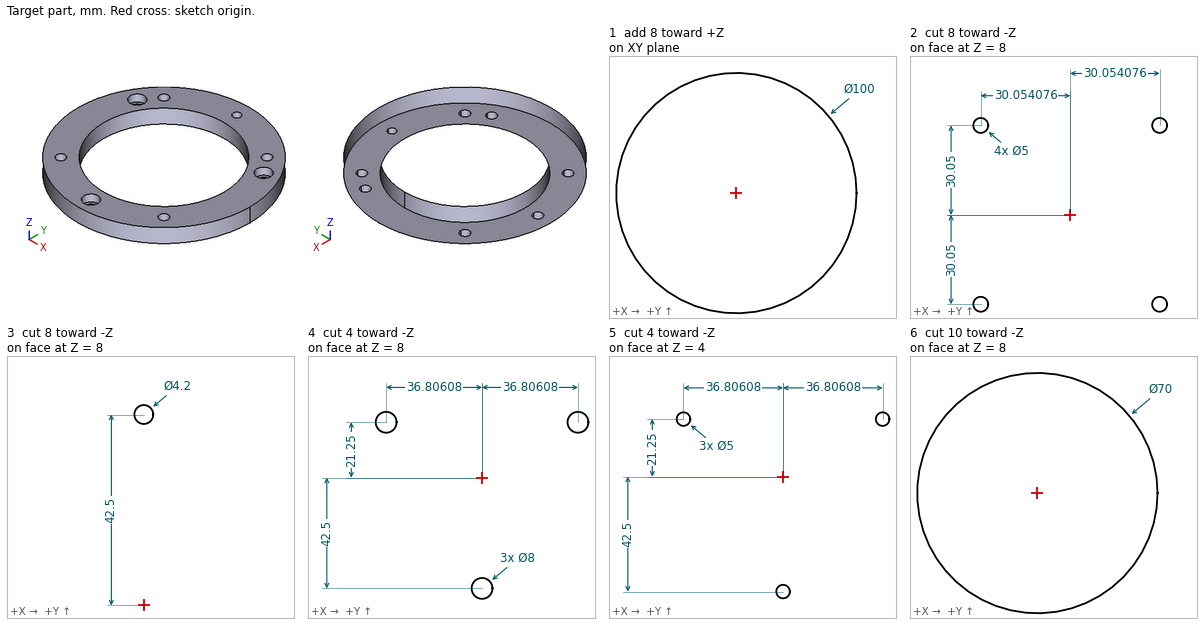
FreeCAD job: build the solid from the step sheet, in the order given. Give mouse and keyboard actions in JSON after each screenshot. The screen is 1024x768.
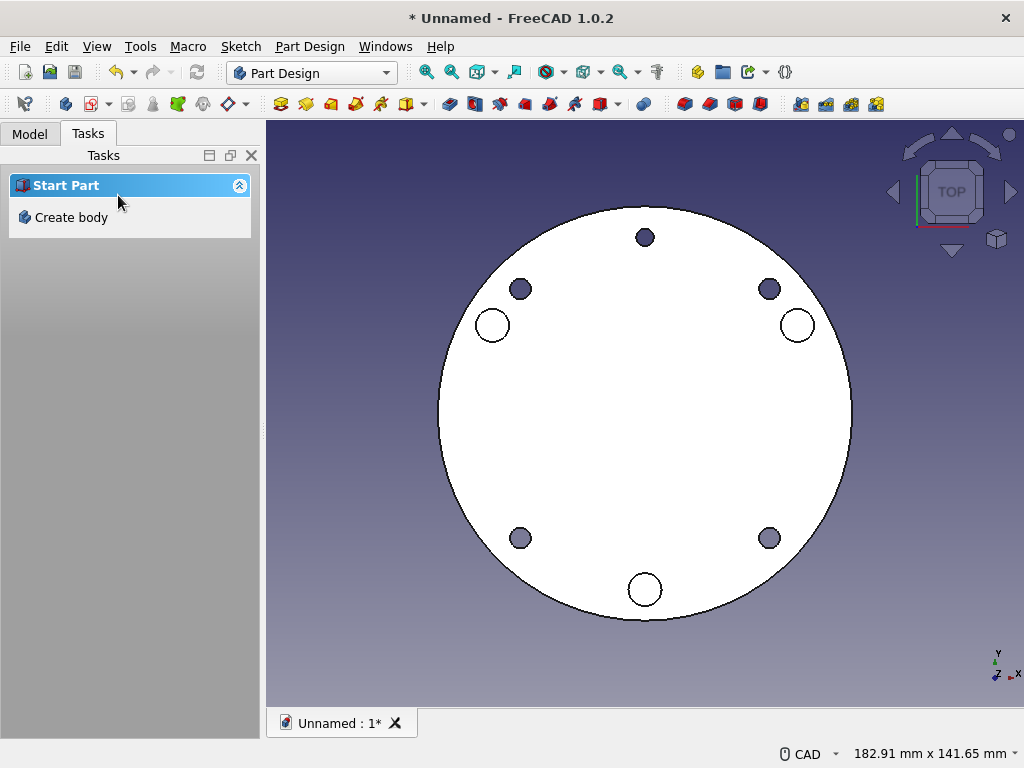
{"action": "left_click", "coordinate": [798, 324]}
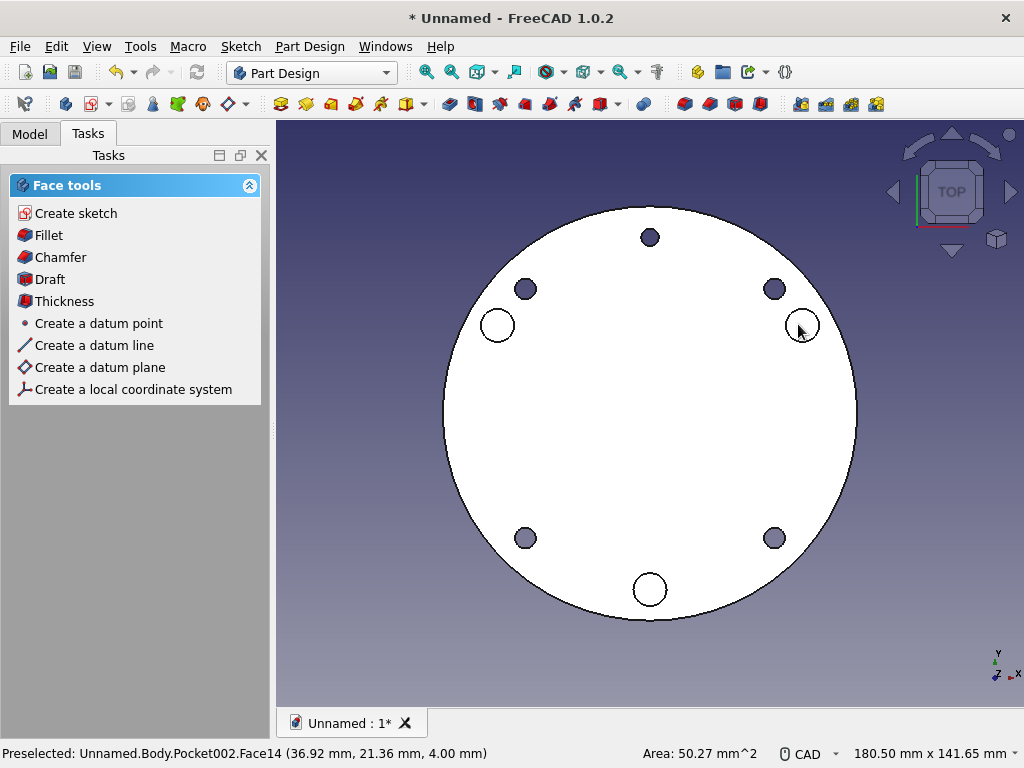
{"action": "left_click", "coordinate": [90, 104]}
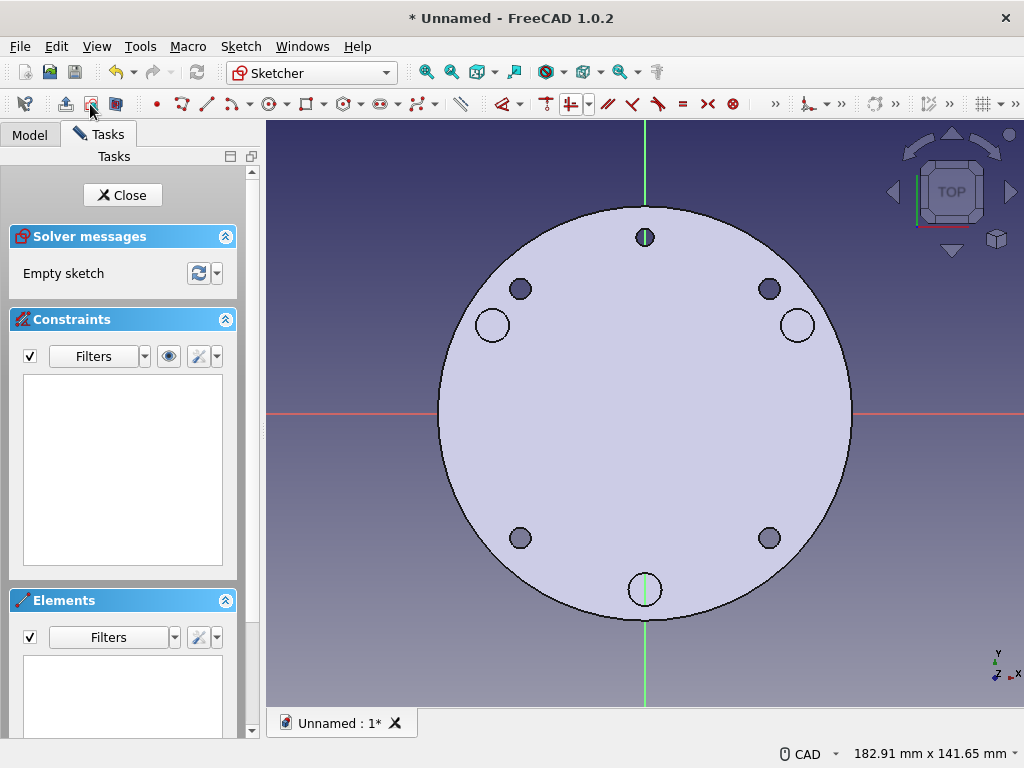
{"action": "left_click", "coordinate": [116, 104]}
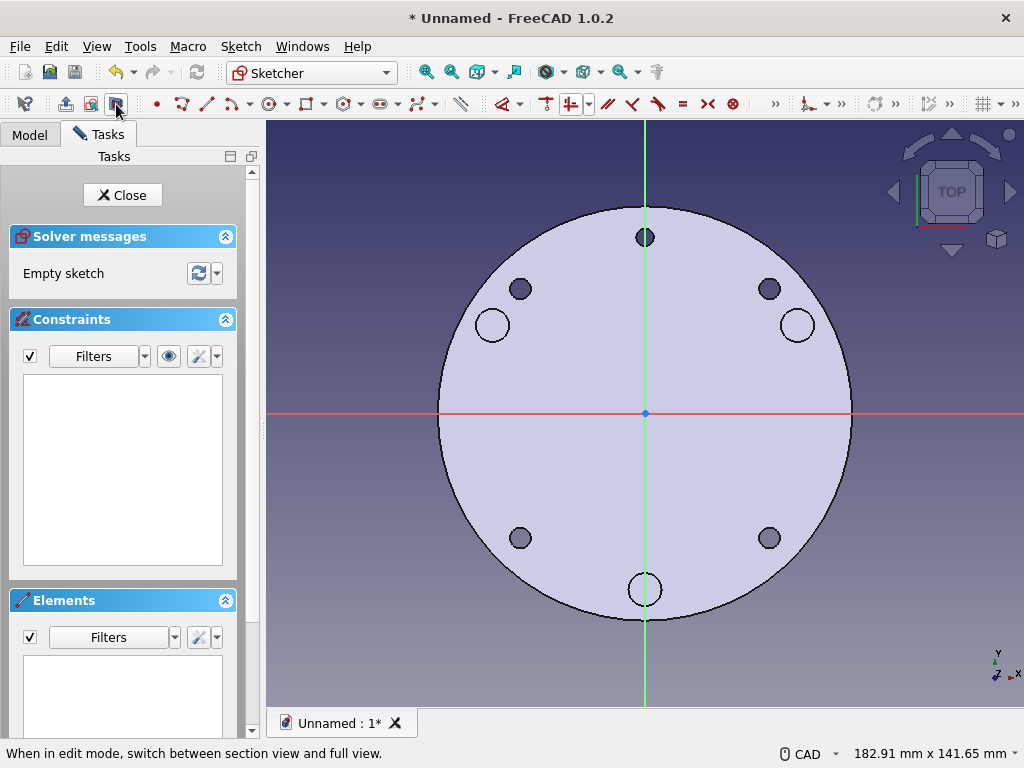
{"action": "left_click", "coordinate": [268, 104]}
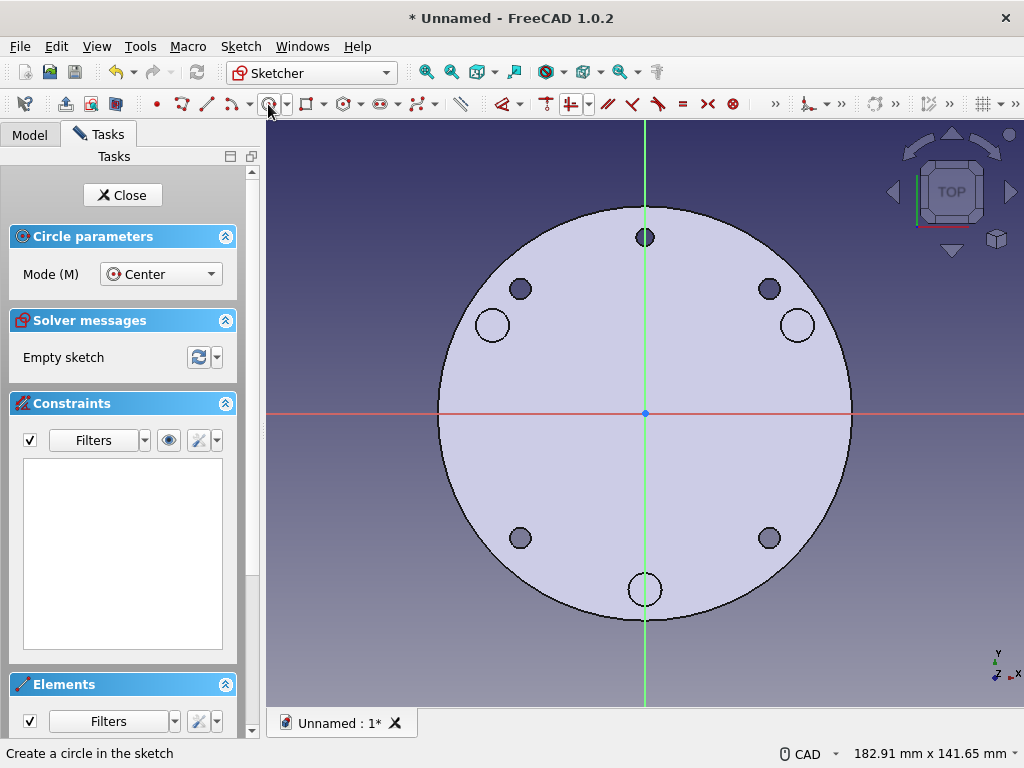
{"action": "scroll", "coordinate": [492, 325], "scroll_direction": "up", "scroll_amount": 4}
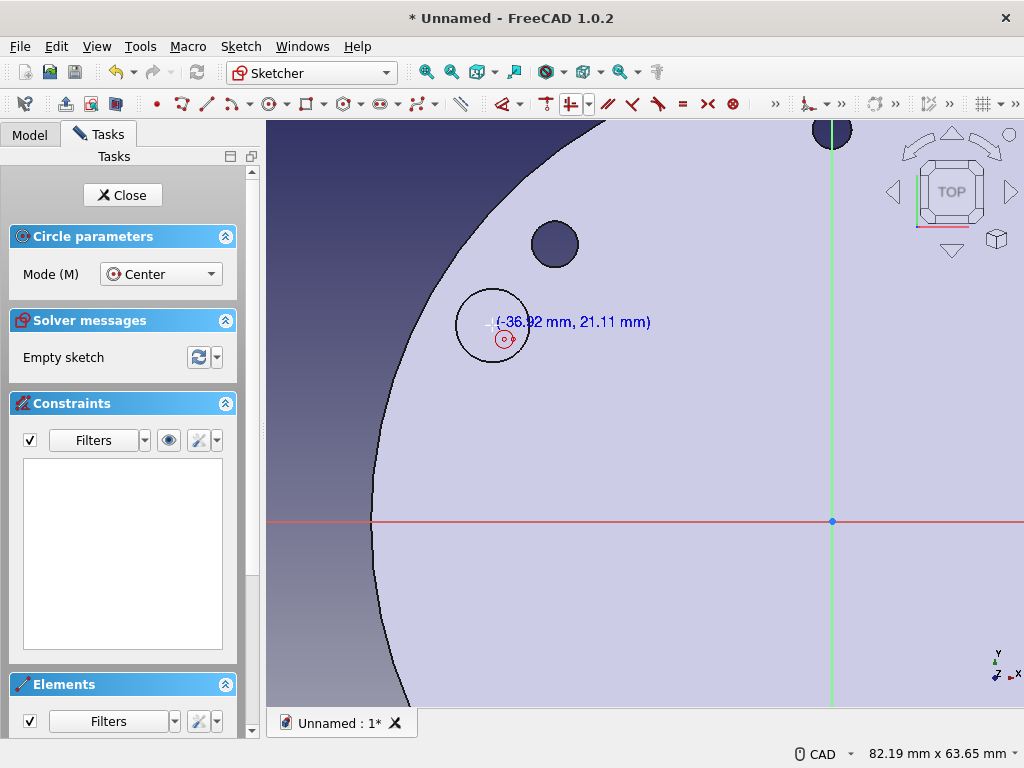
{"action": "left_click", "coordinate": [493, 326]}
{"action": "mouse_move", "coordinate": [509, 309]}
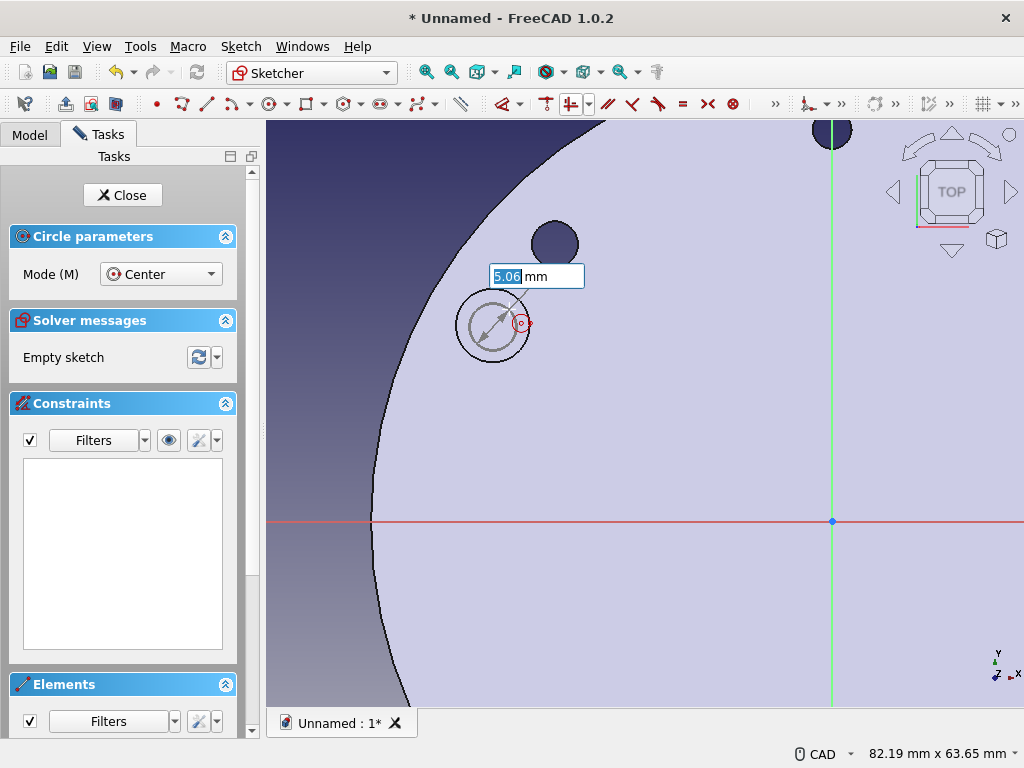
{"action": "type", "text": "5"}
{"action": "key", "text": "Return"}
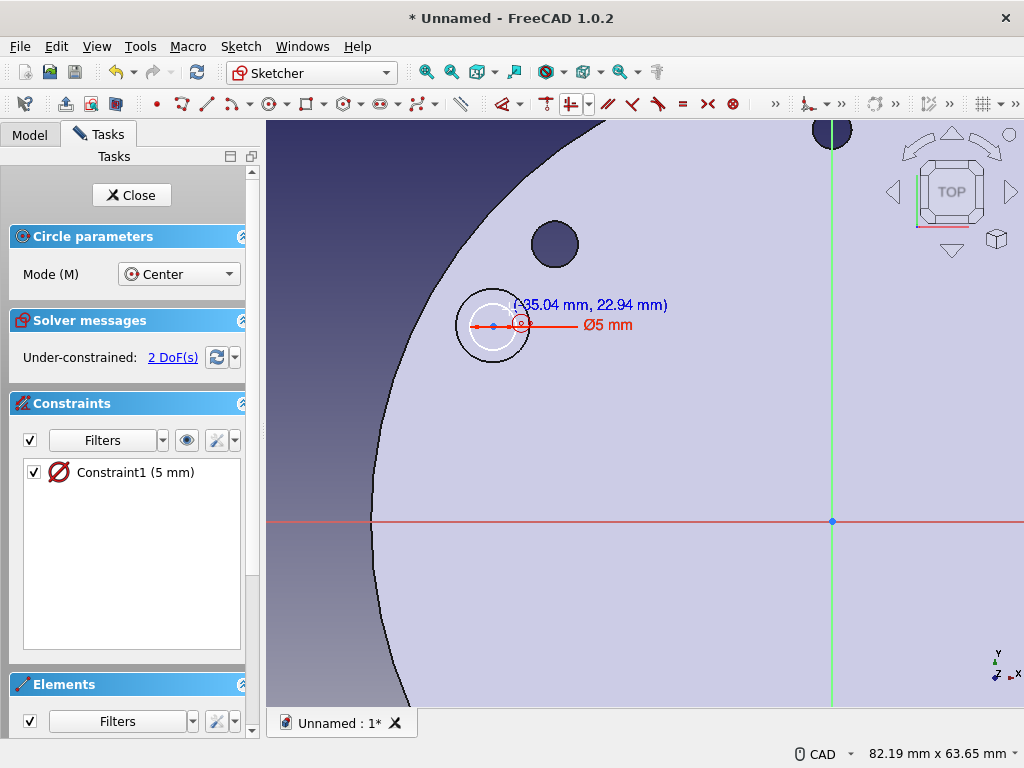
{"action": "scroll", "coordinate": [294, 163], "scroll_direction": "down", "scroll_amount": 3}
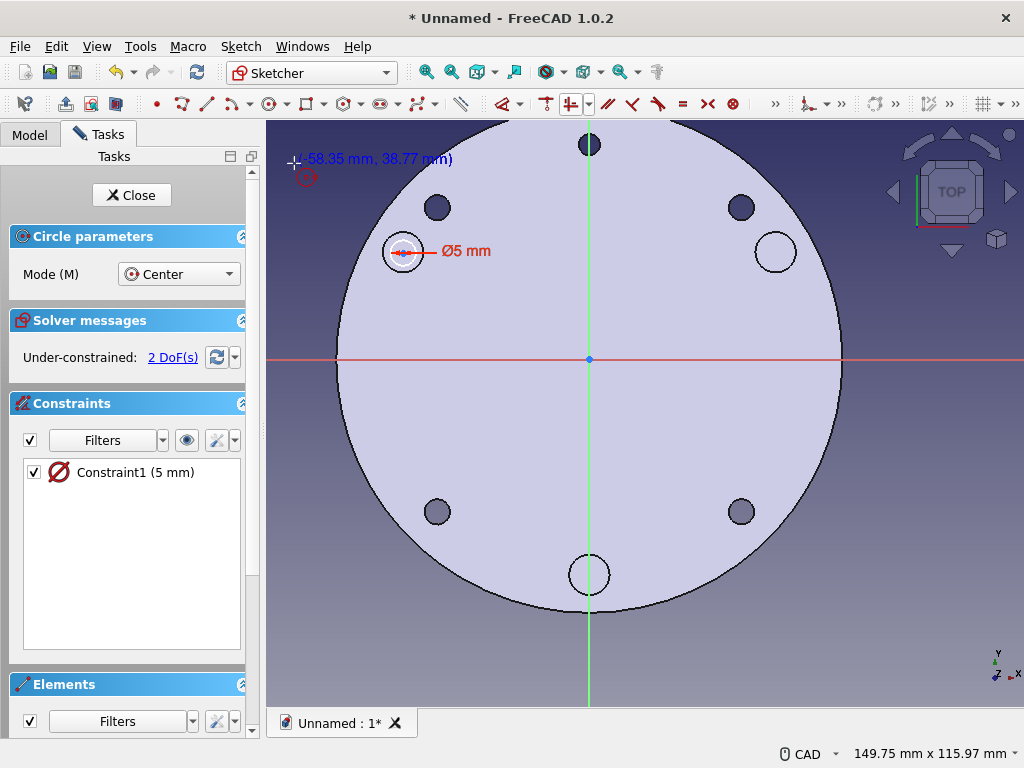
{"action": "scroll", "coordinate": [589, 575], "scroll_direction": "up", "scroll_amount": 3}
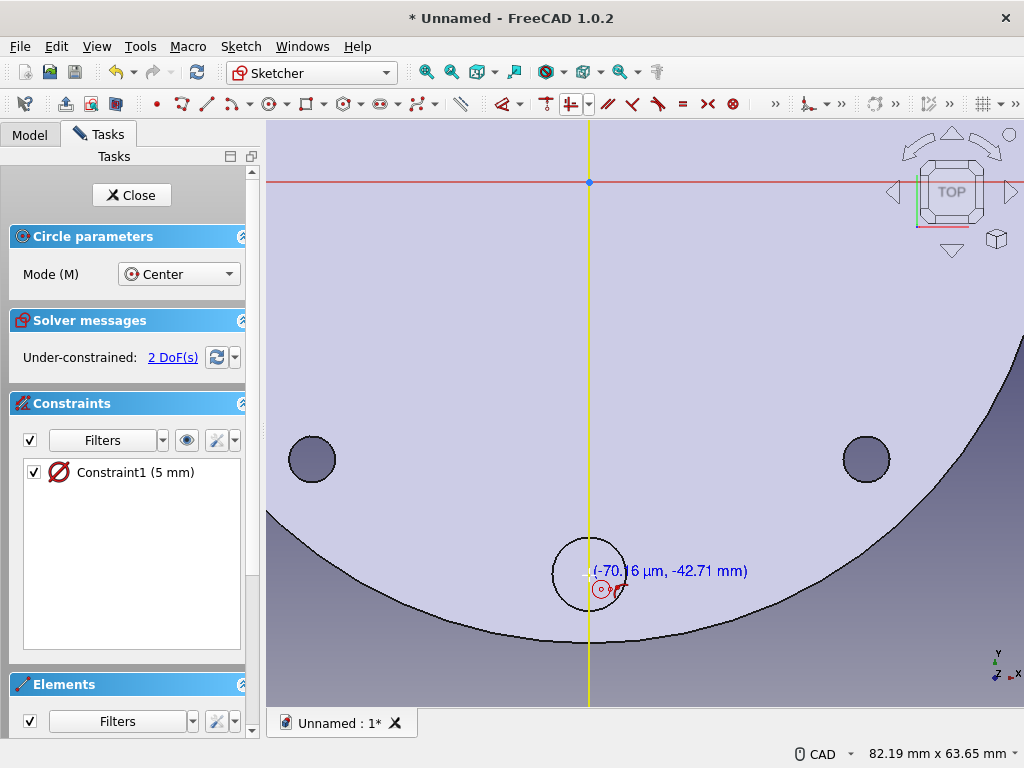
{"action": "left_click", "coordinate": [589, 574]}
{"action": "mouse_move", "coordinate": [606, 558]}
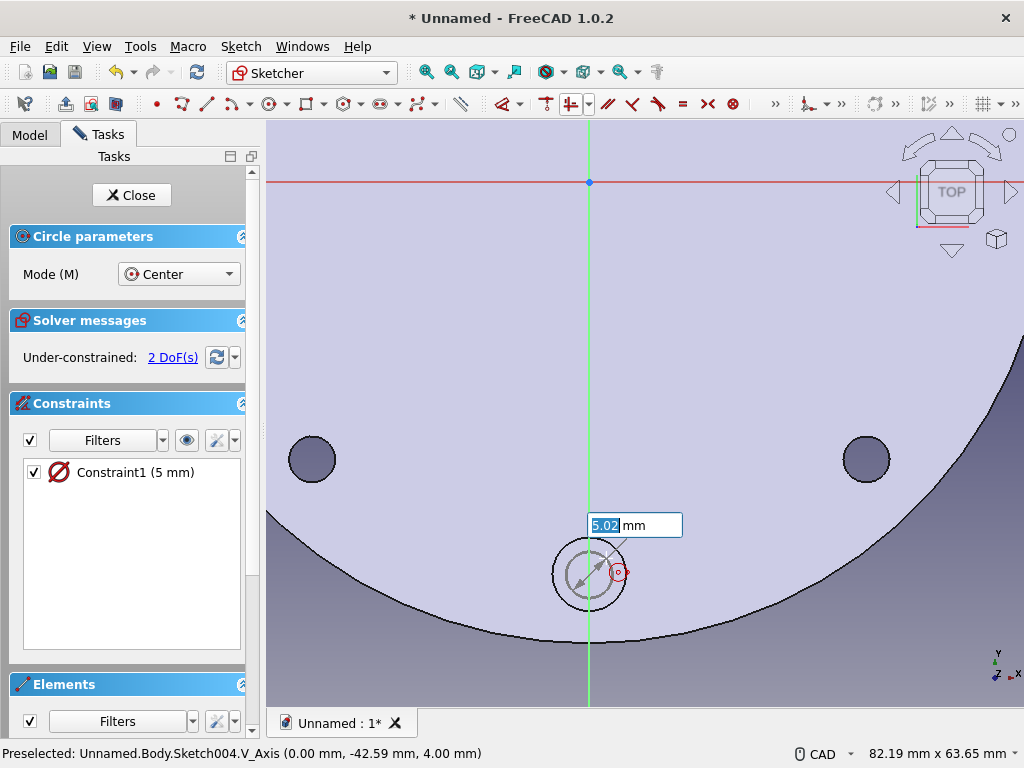
{"action": "type", "text": "5"}
{"action": "key", "text": "Return"}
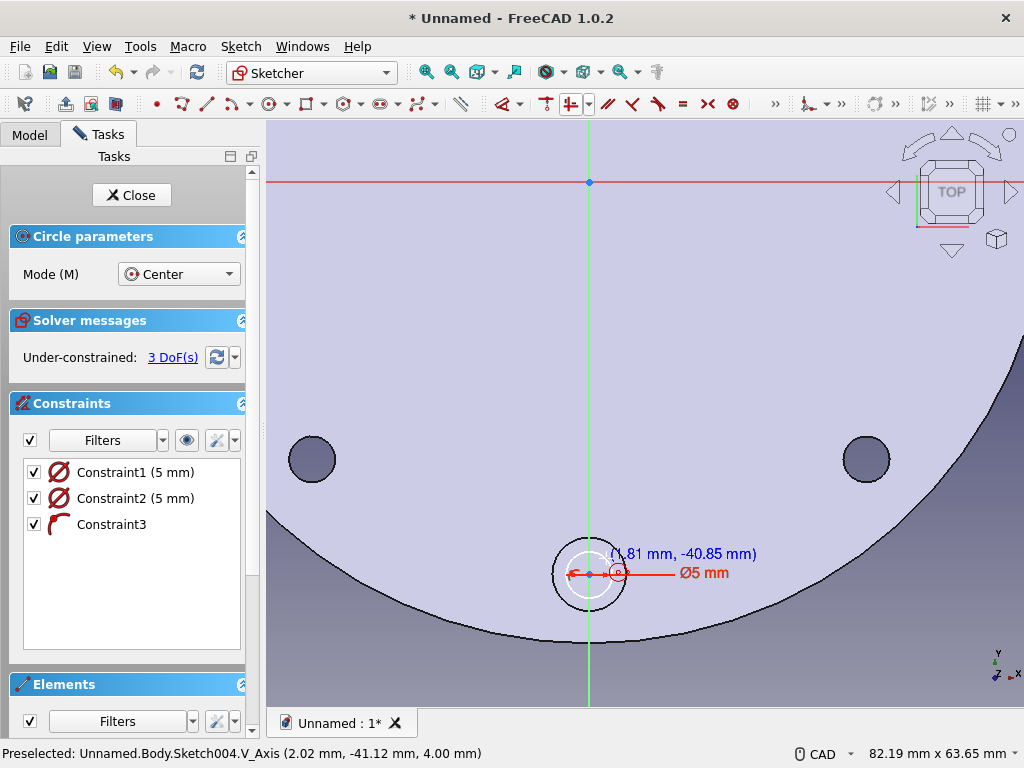
{"action": "scroll", "coordinate": [561, 576], "scroll_direction": "down", "scroll_amount": 3}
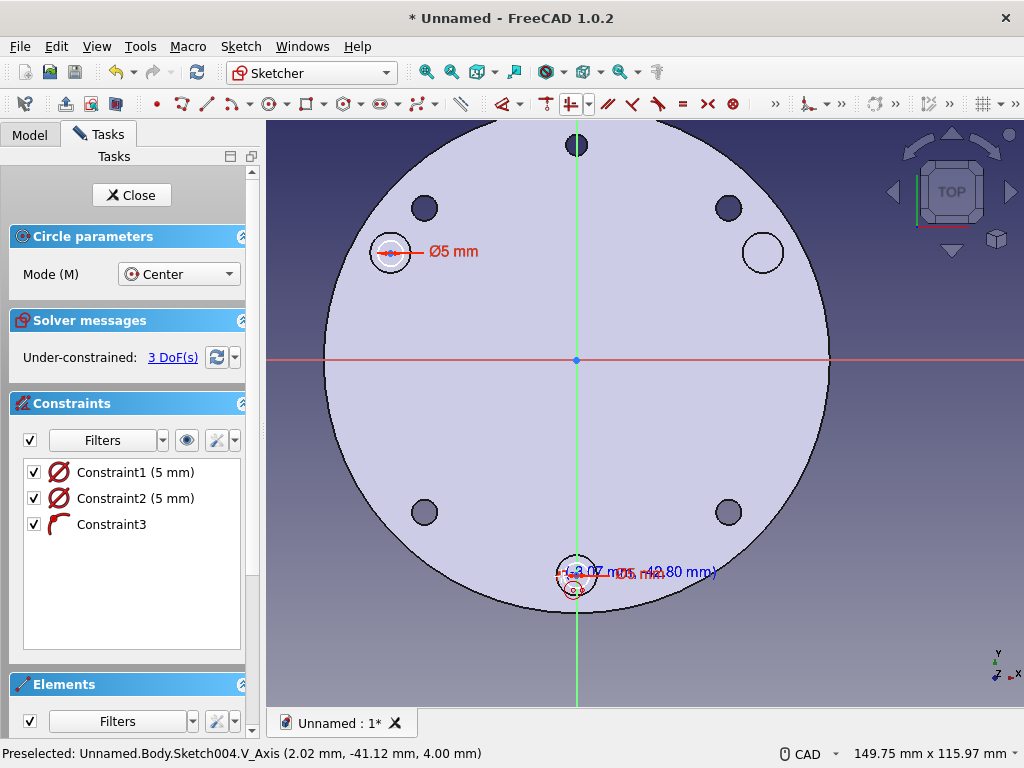
{"action": "scroll", "coordinate": [763, 253], "scroll_direction": "up", "scroll_amount": 3}